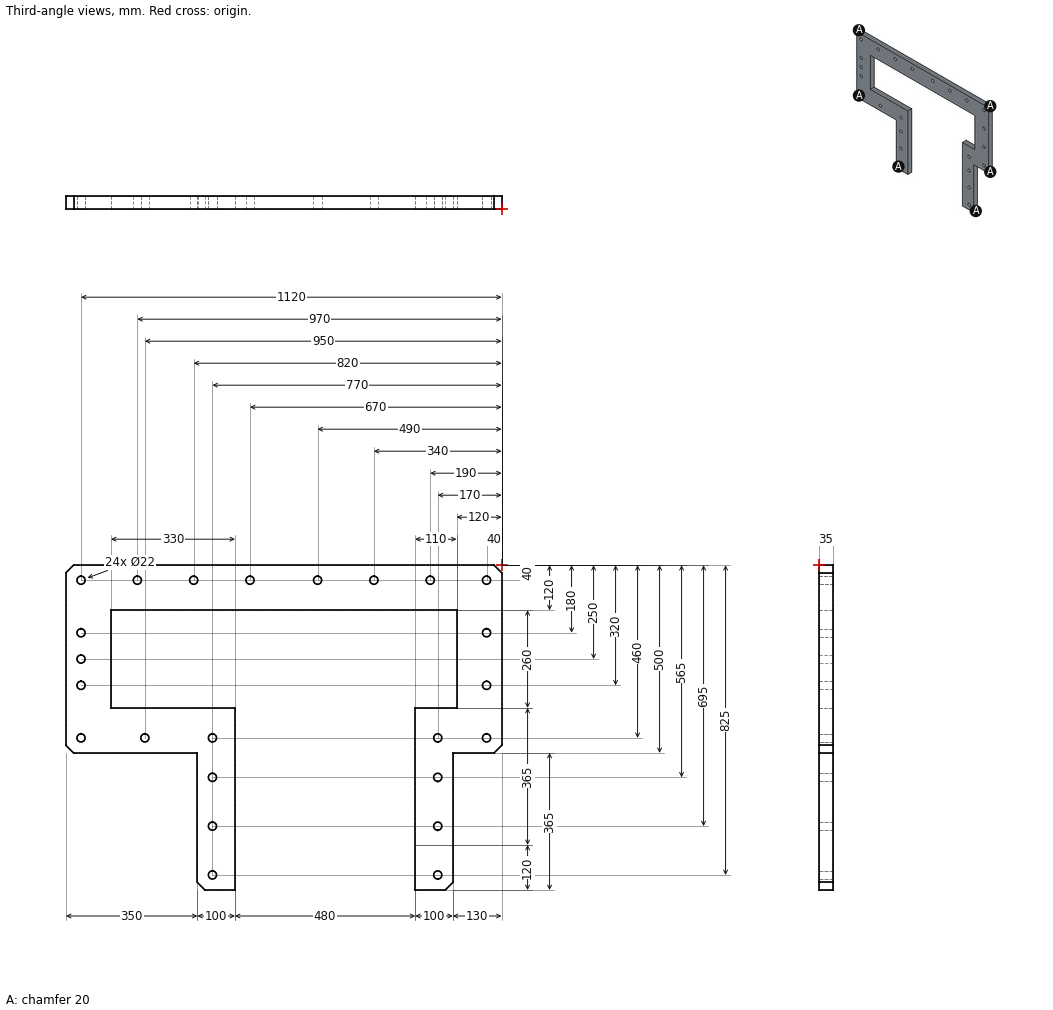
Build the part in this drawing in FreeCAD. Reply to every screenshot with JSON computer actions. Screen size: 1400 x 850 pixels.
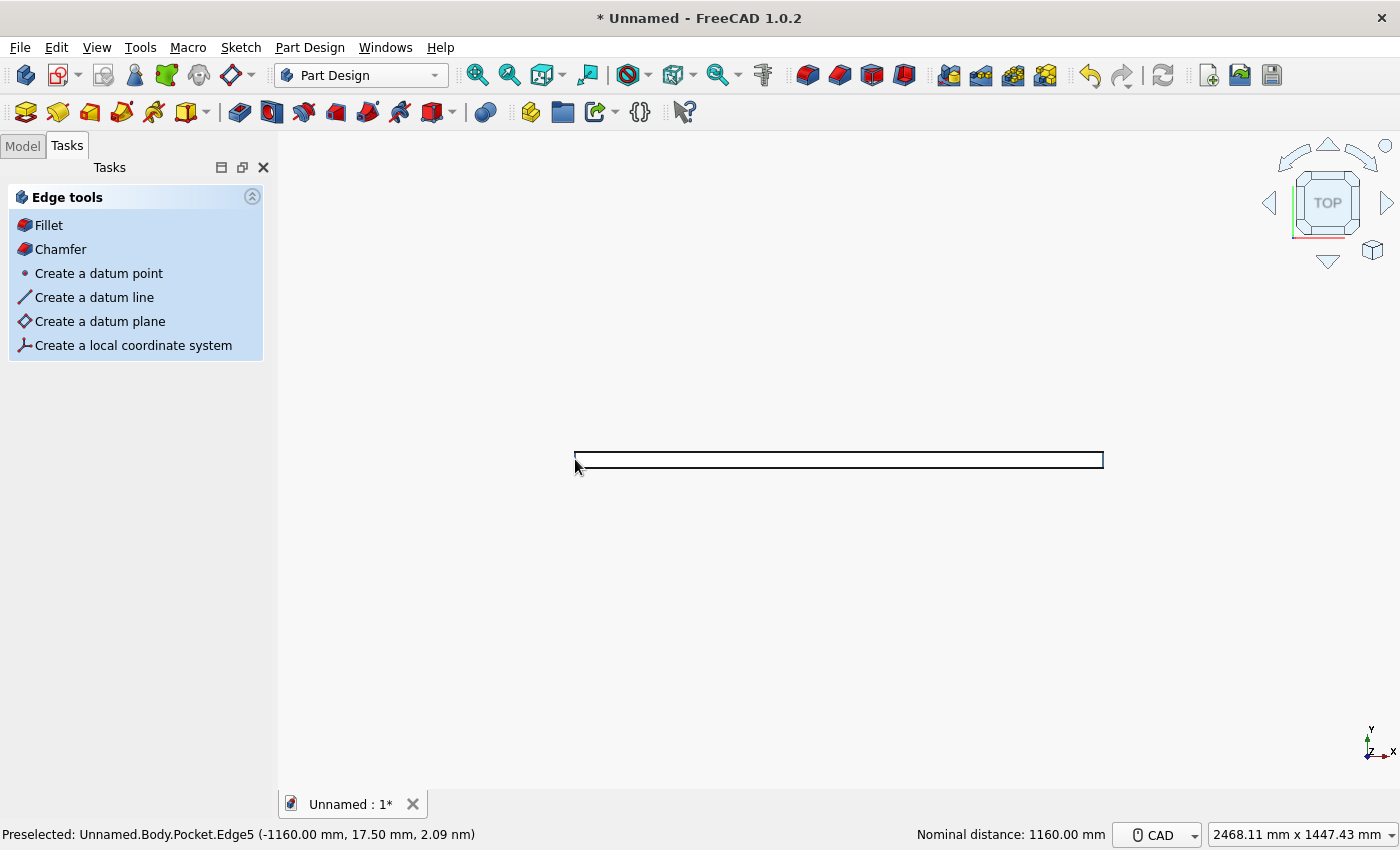
{"action": "scroll", "coordinate": [575, 459], "scroll_direction": "up", "scroll_amount": 5}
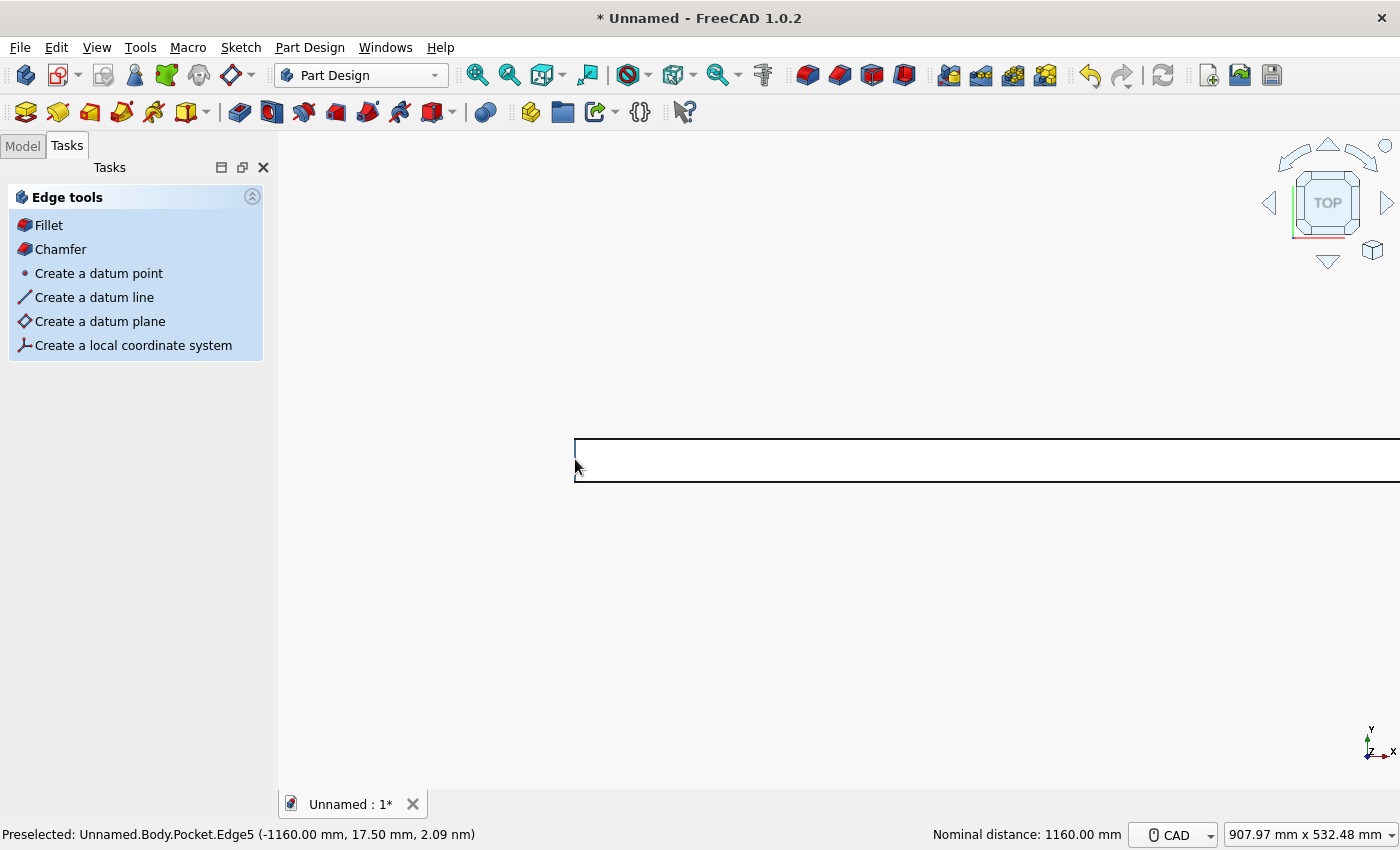
{"action": "key", "text": "v f"}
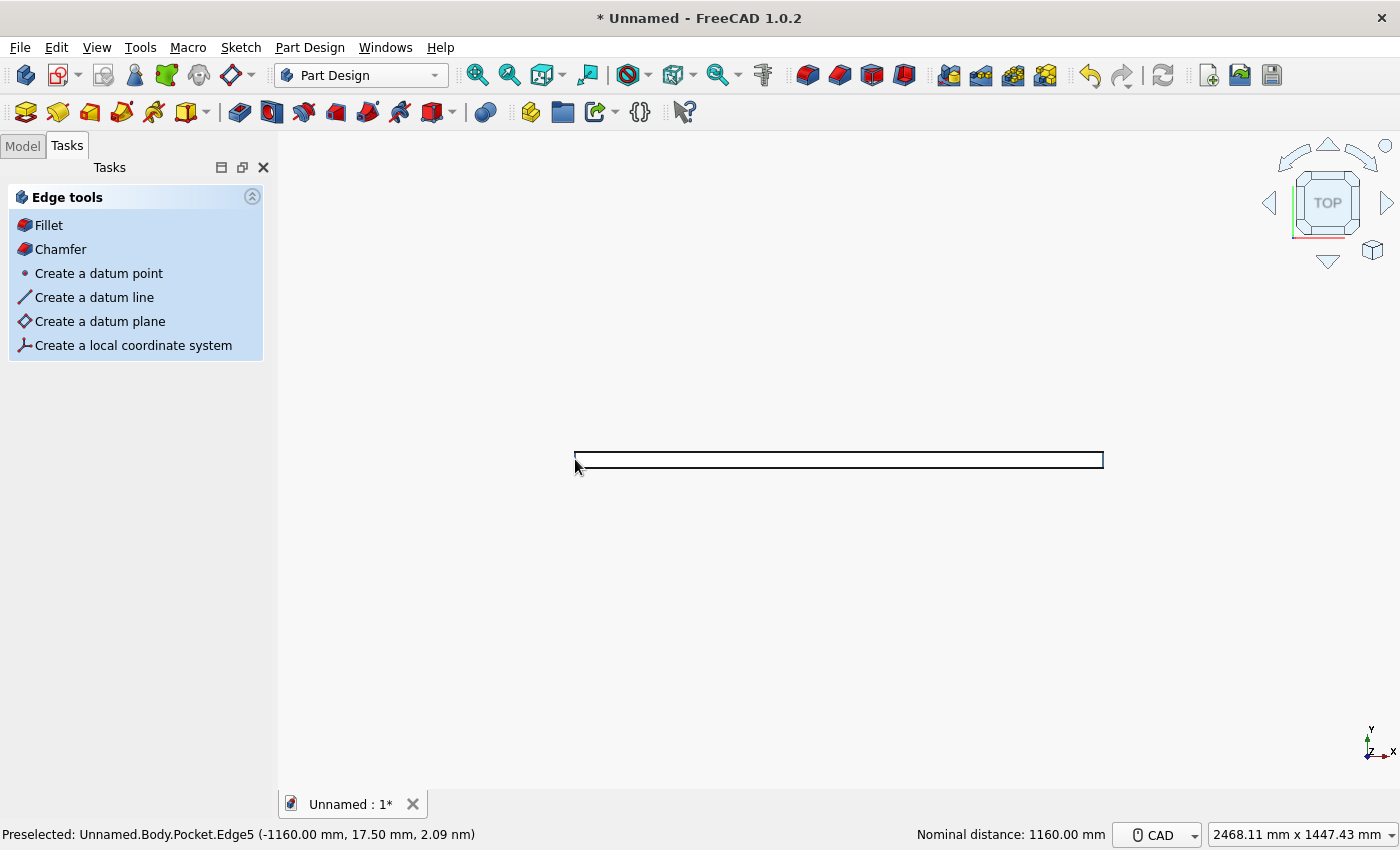
{"action": "key", "text": "1"}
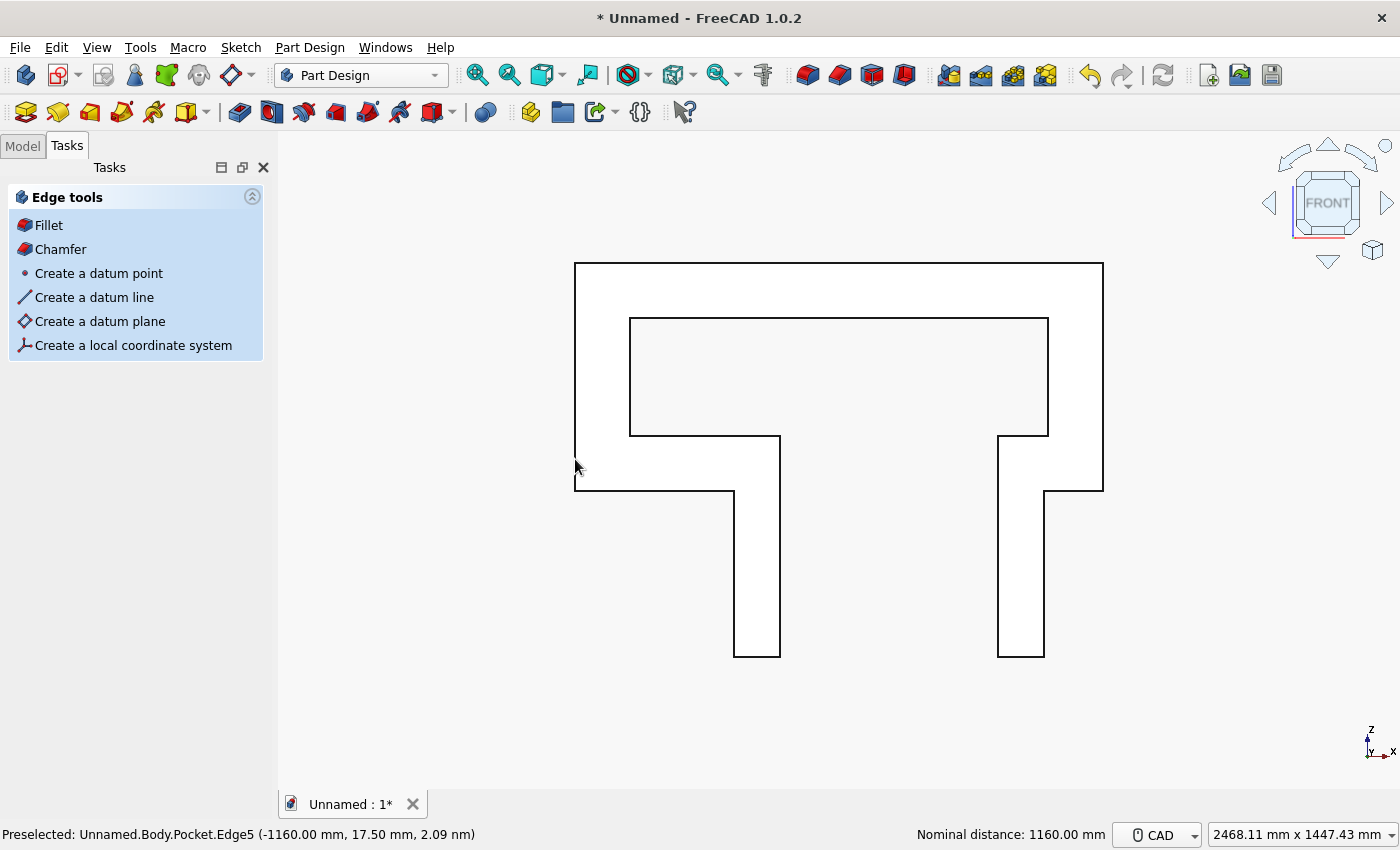
{"action": "scroll", "coordinate": [575, 490], "scroll_direction": "up", "scroll_amount": 5}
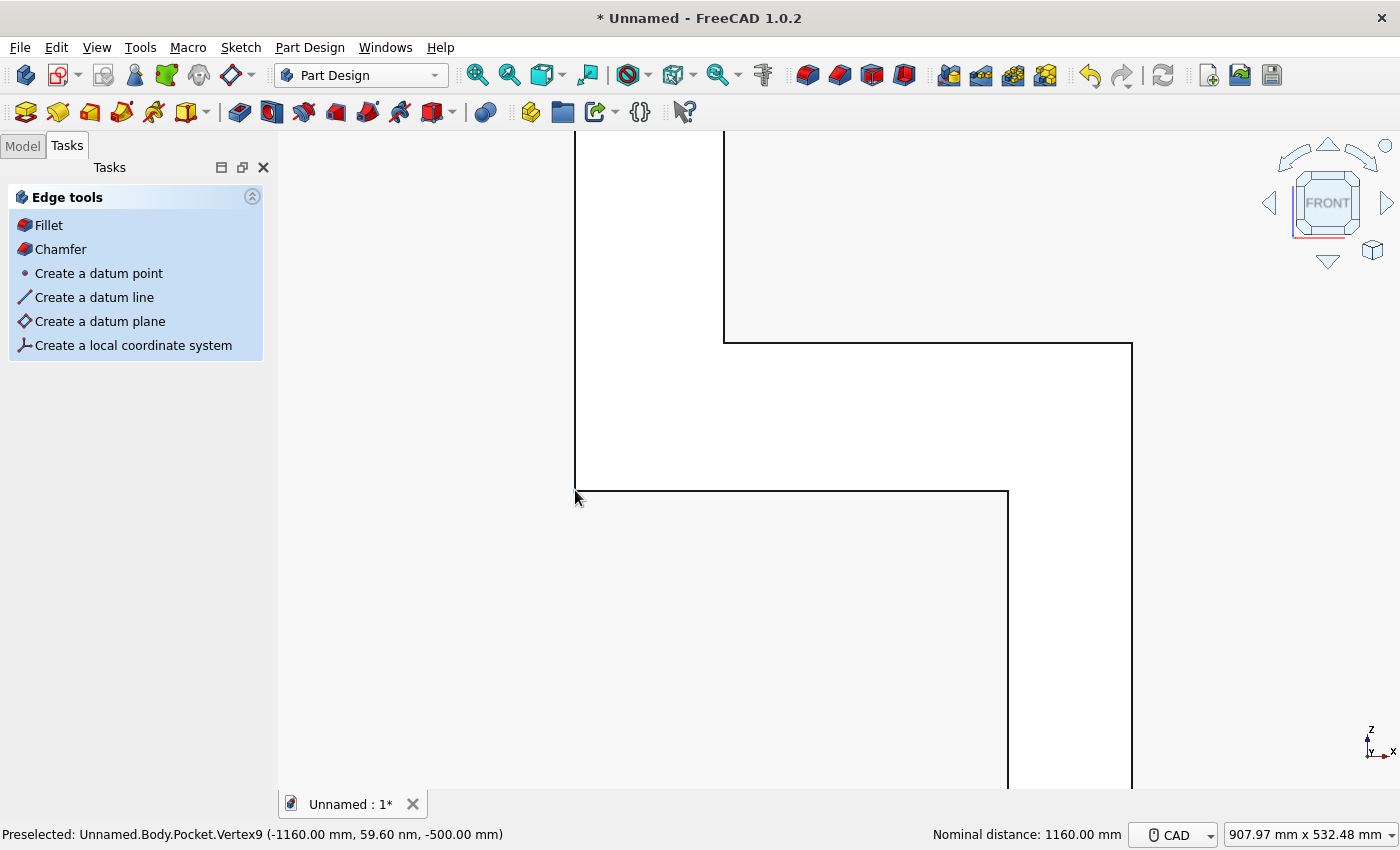
{"action": "key", "text": "v f"}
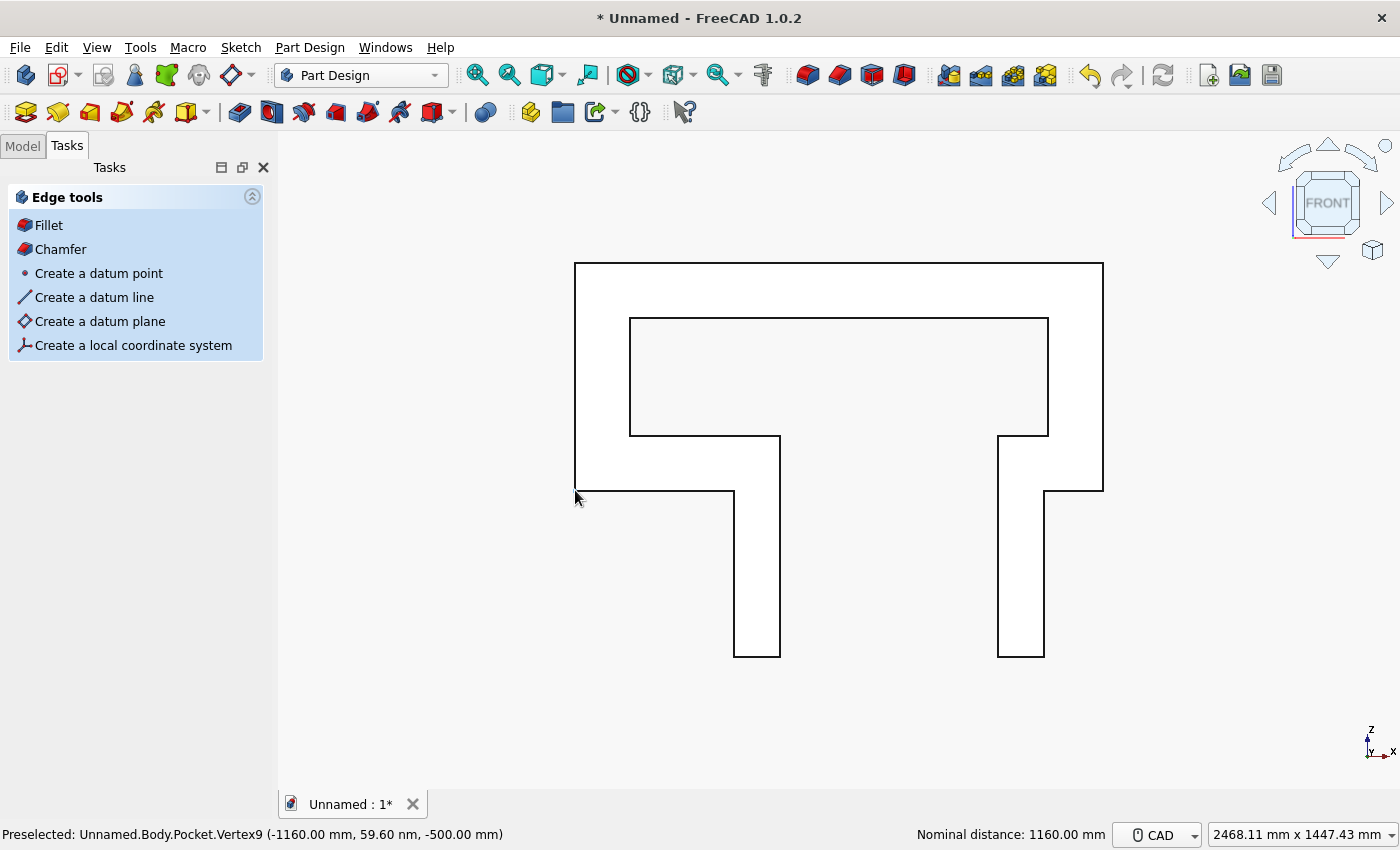
{"action": "key", "text": "3"}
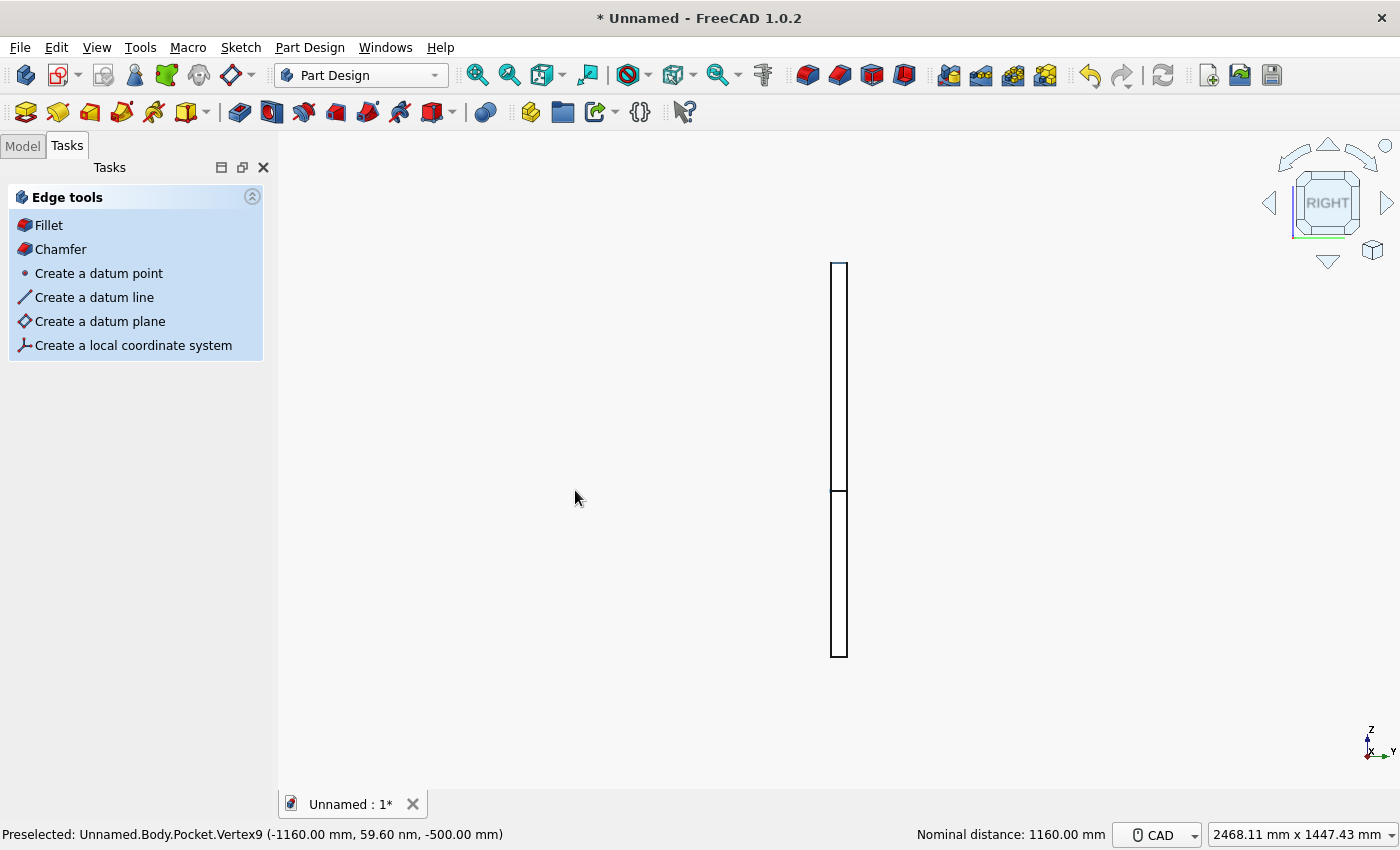
{"action": "left_click", "coordinate": [839, 656], "text": "ctrl"}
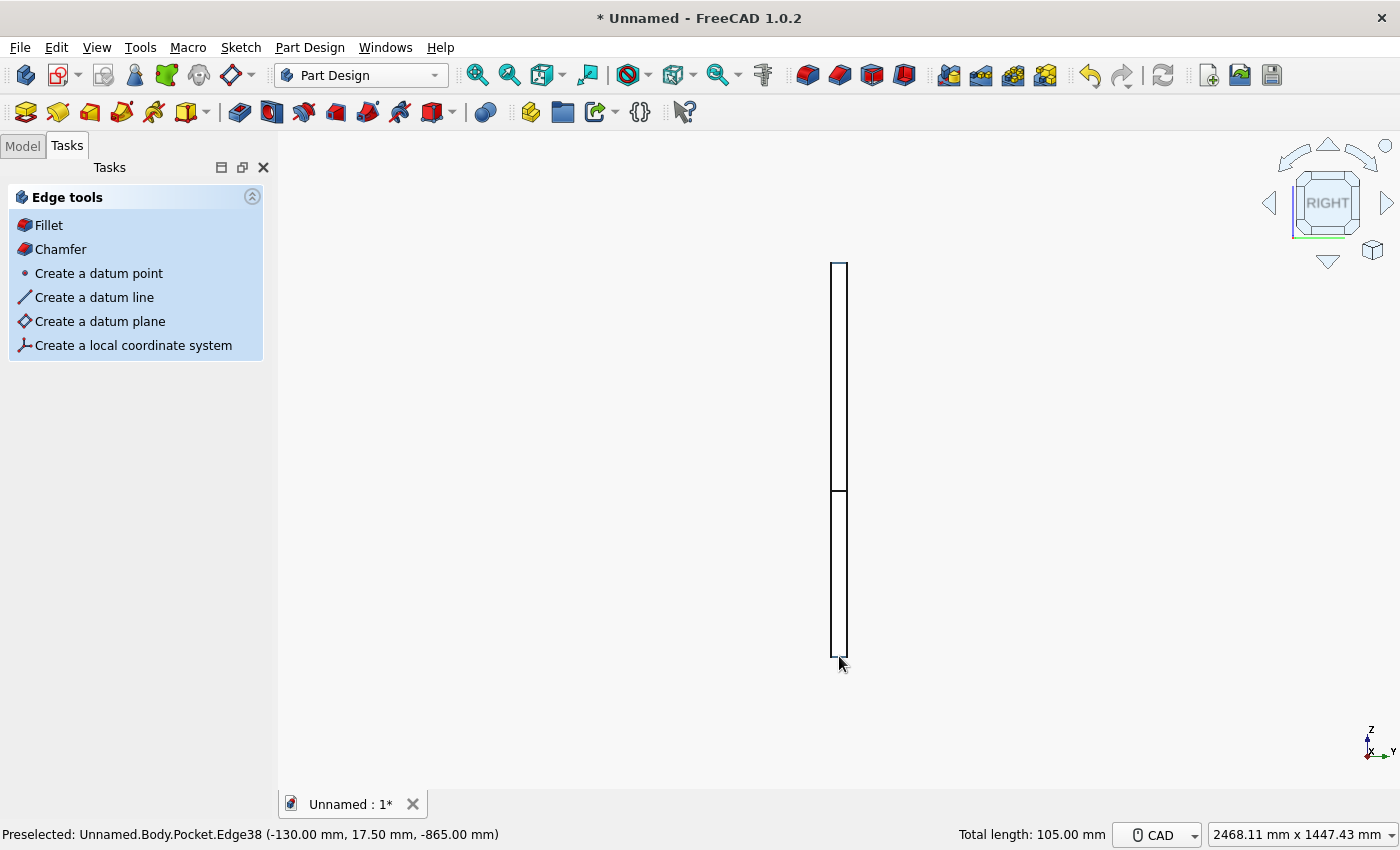
{"action": "left_click", "coordinate": [839, 490], "text": "ctrl"}